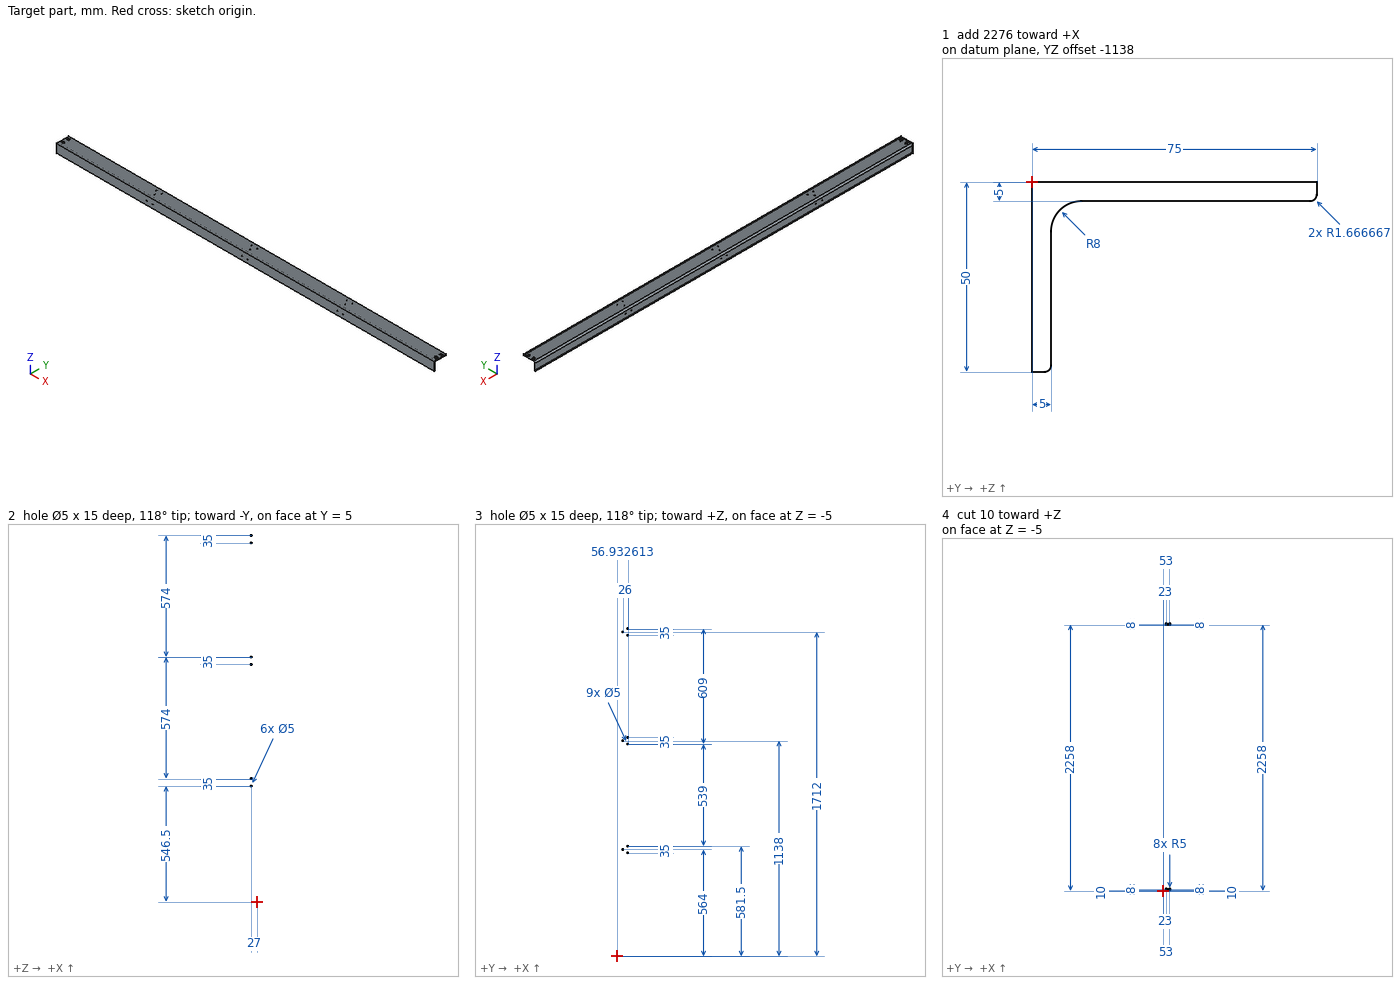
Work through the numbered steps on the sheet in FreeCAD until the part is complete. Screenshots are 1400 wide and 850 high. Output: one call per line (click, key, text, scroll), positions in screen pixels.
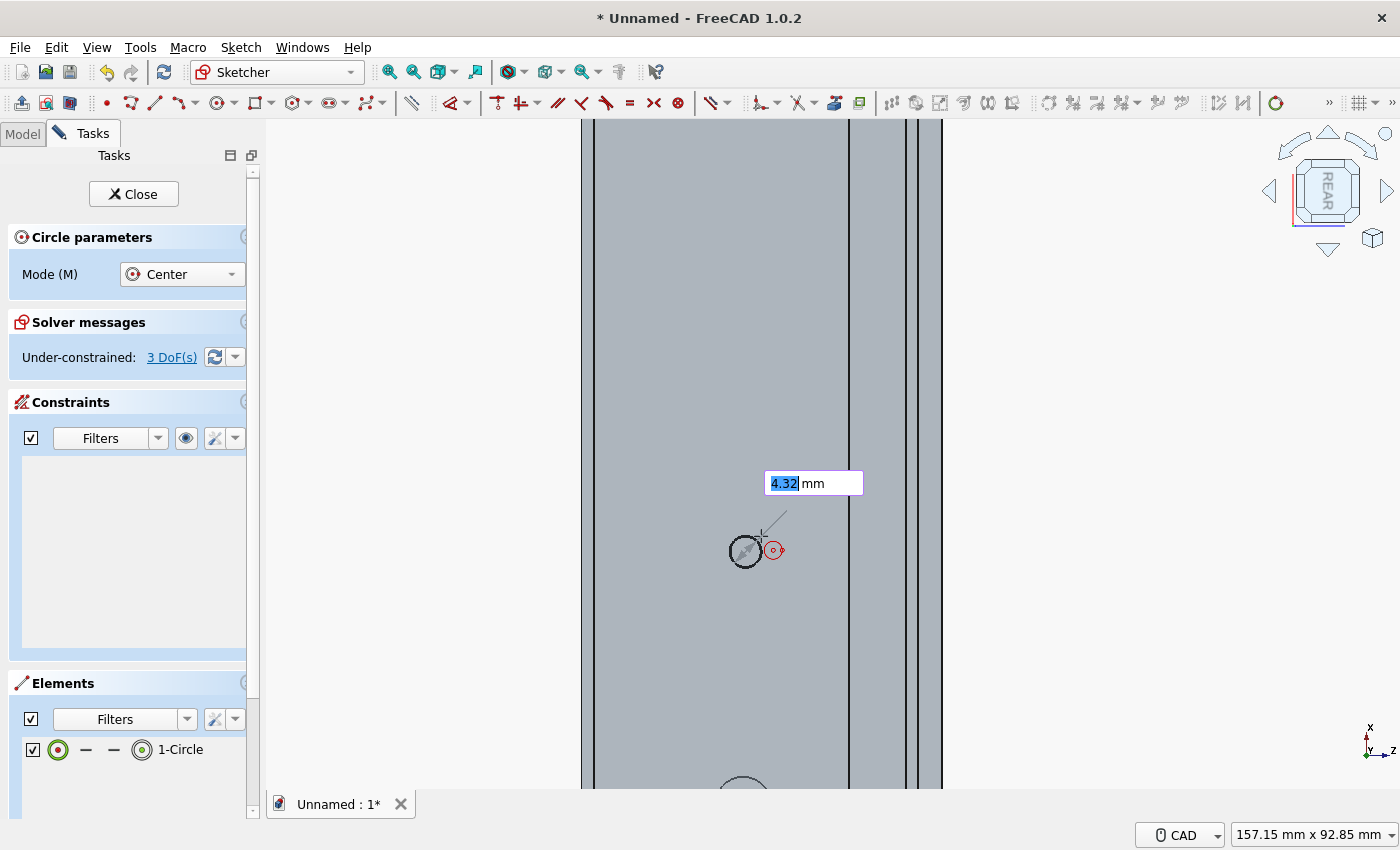
click(760, 530)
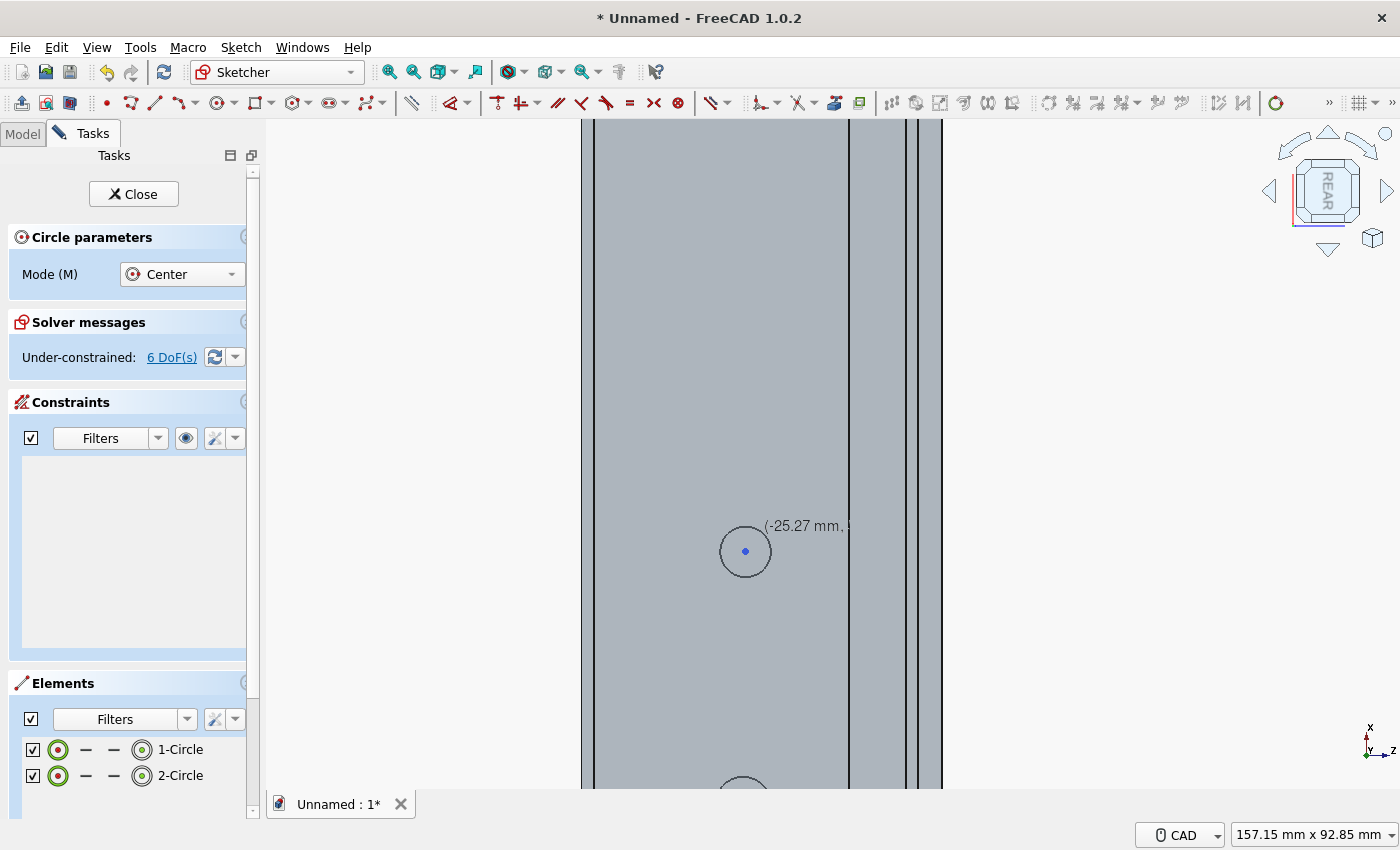
scroll(761, 537, down, 16)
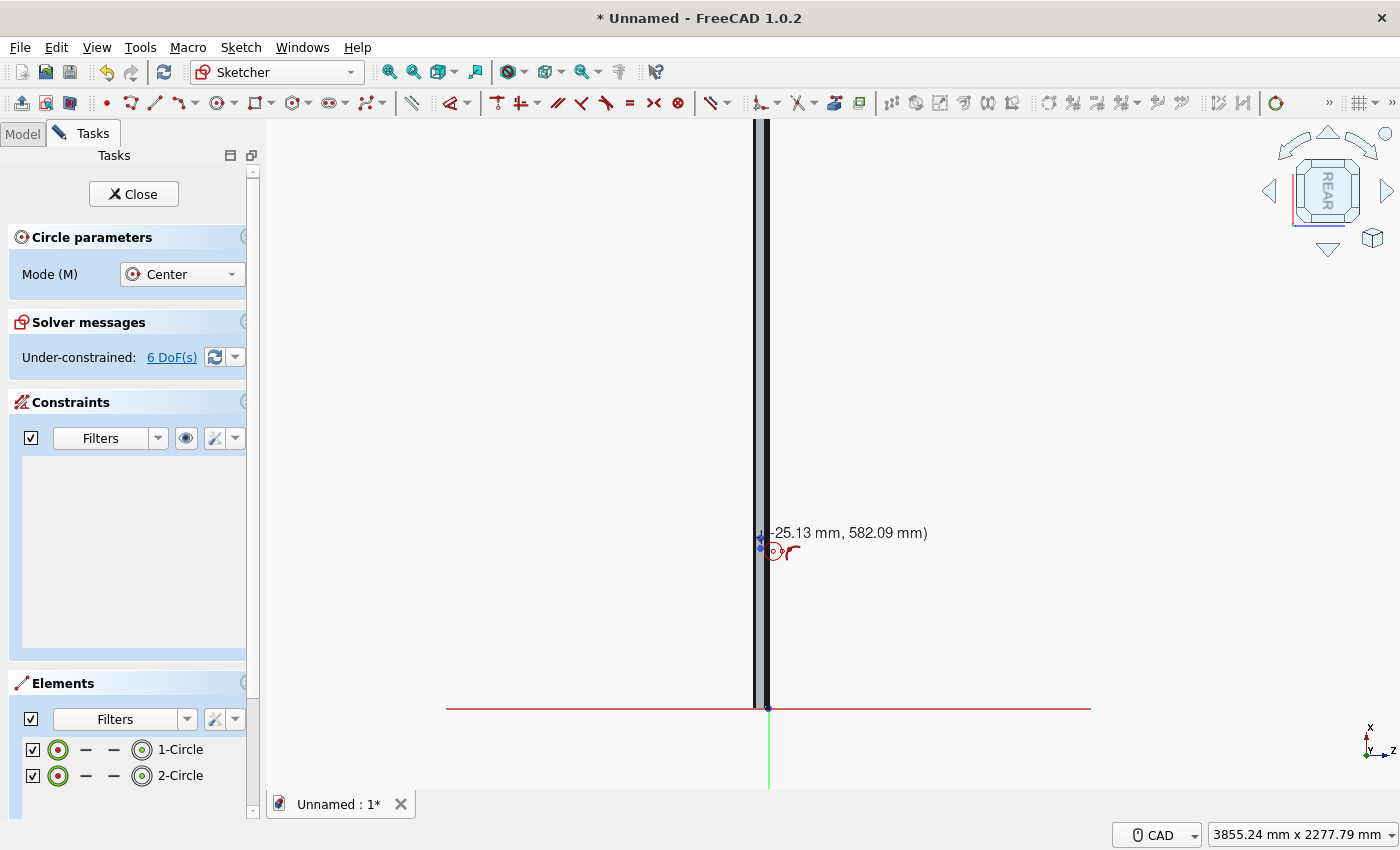
scroll(761, 369, up, 18)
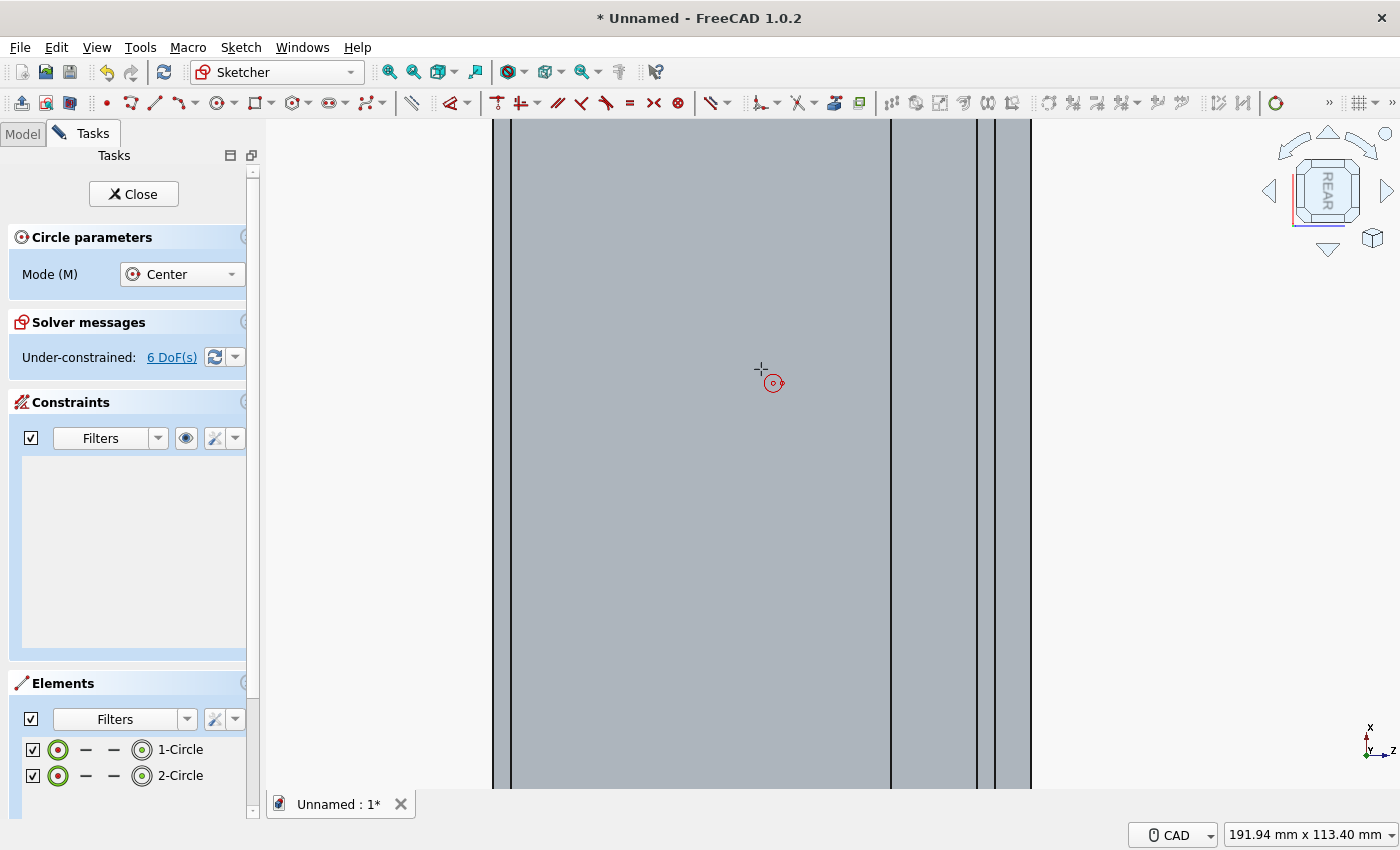
scroll(761, 369, down, 18)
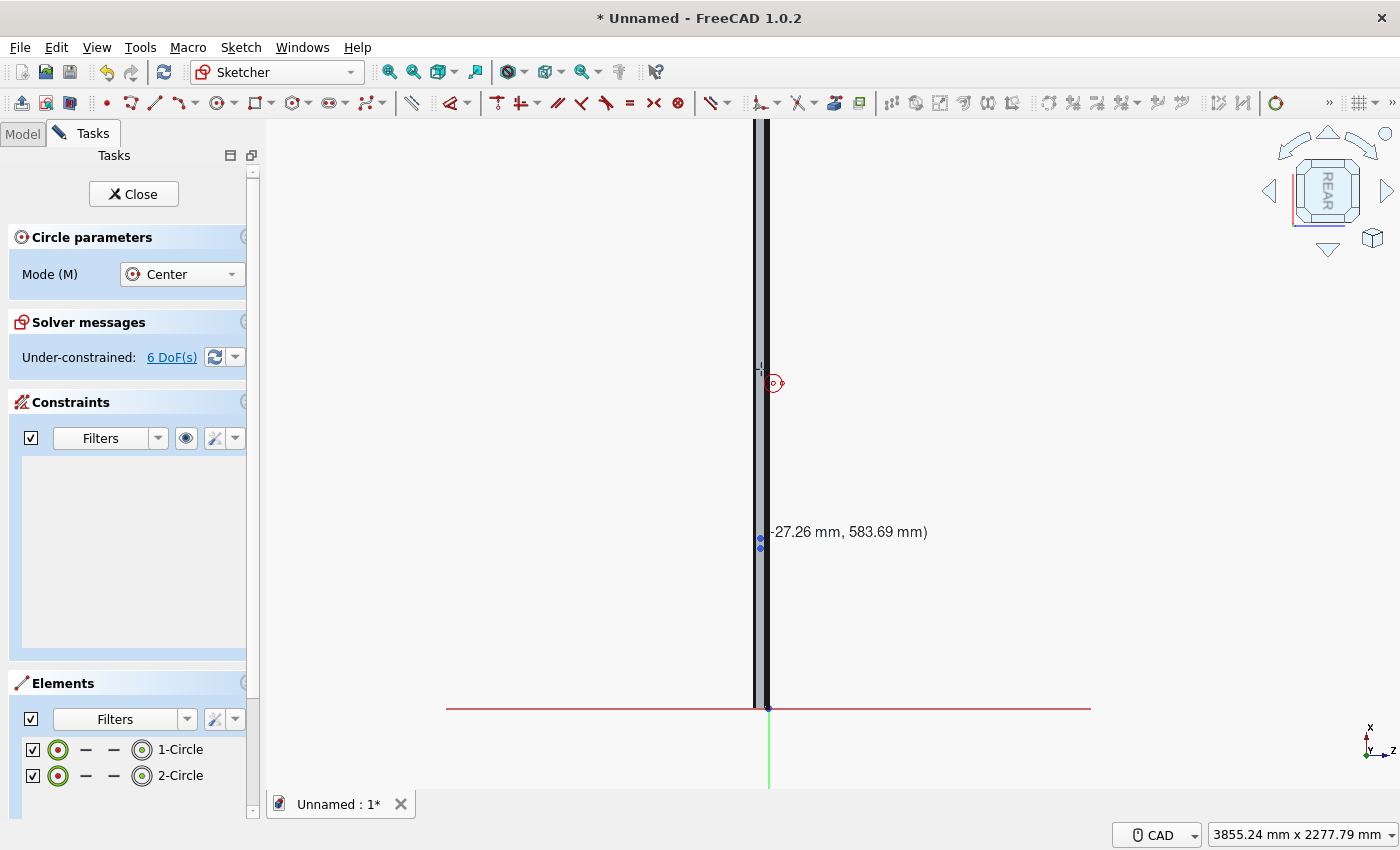
scroll(761, 369, up, 4)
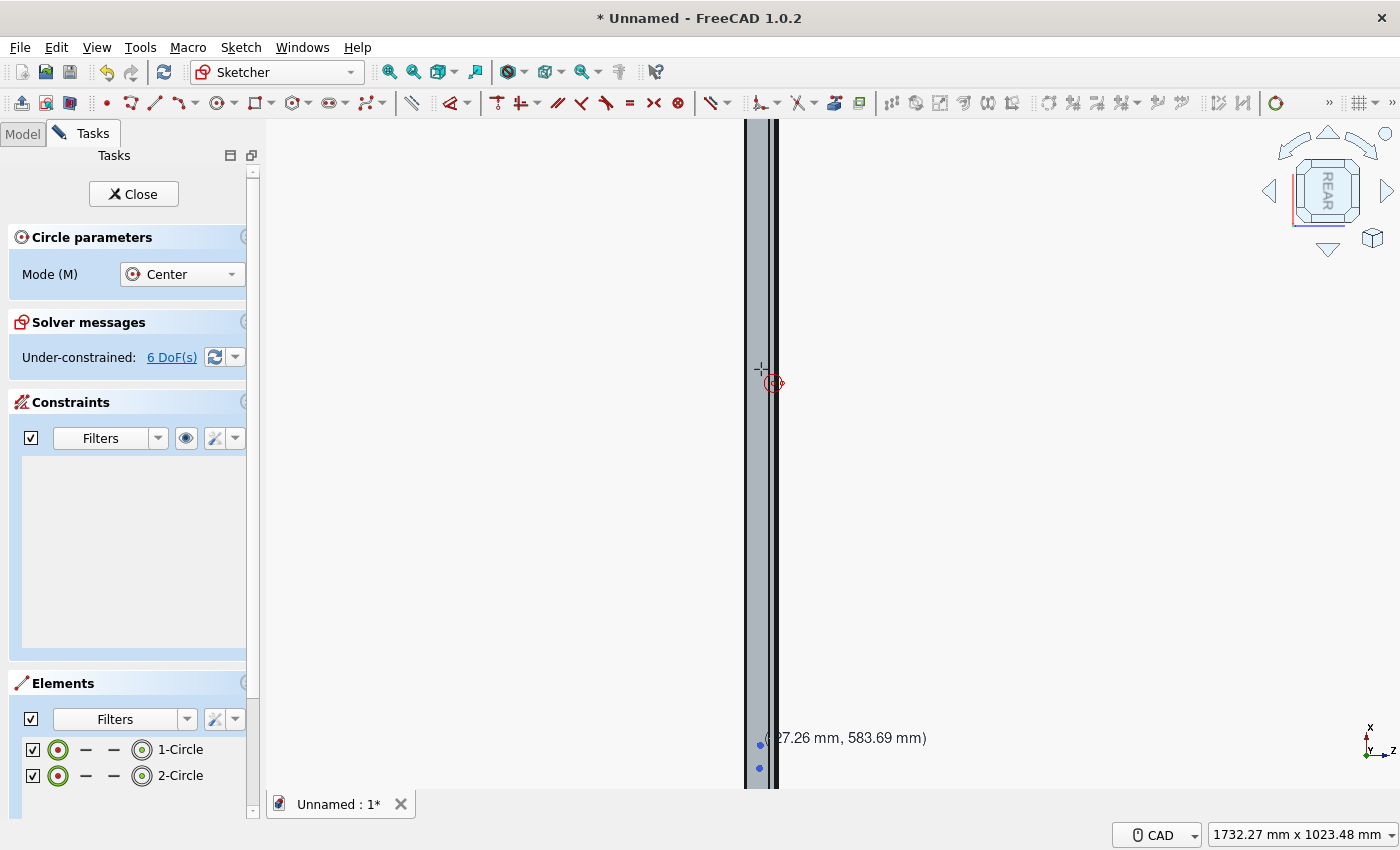
click(760, 368)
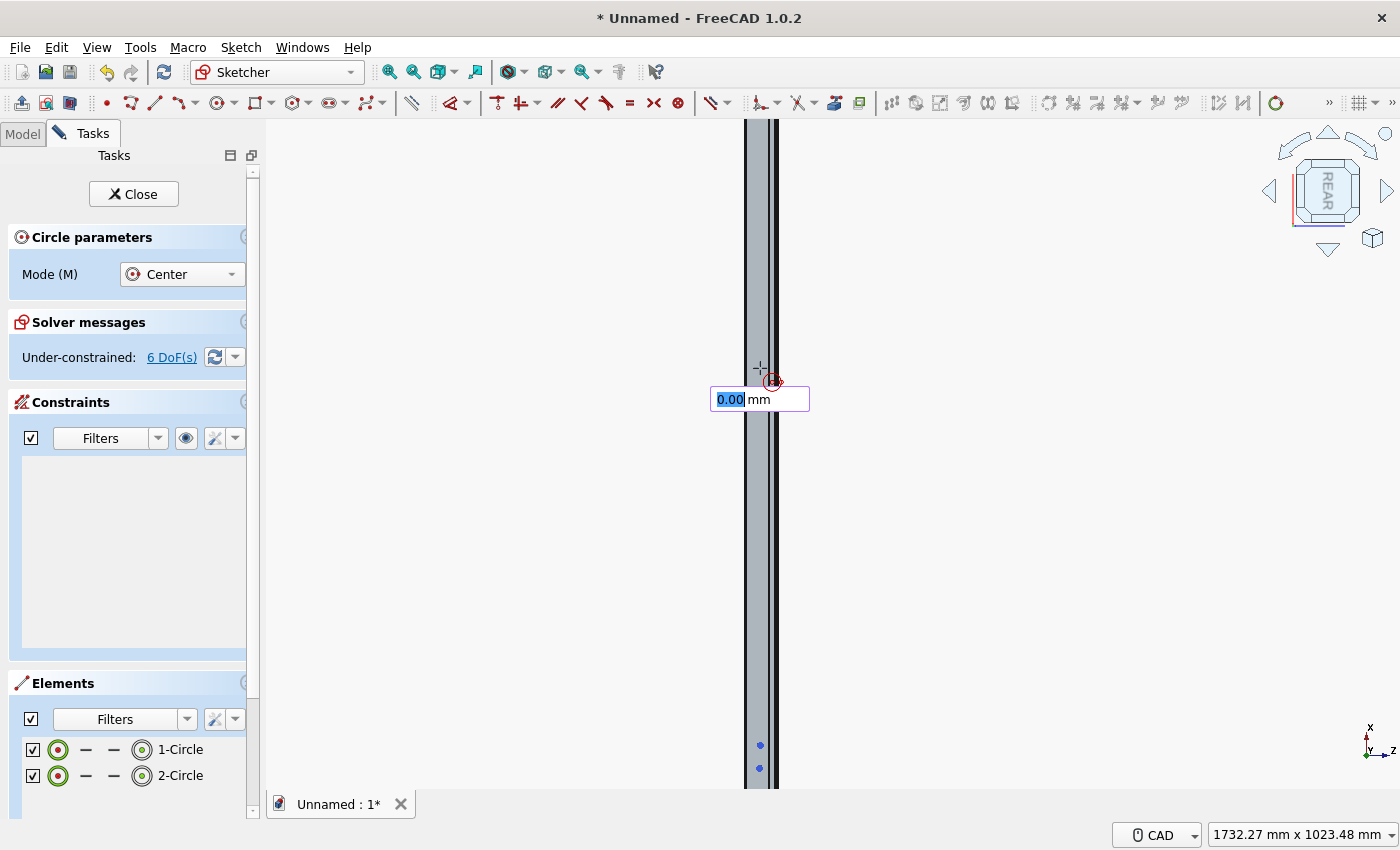
scroll(761, 367, up, 12)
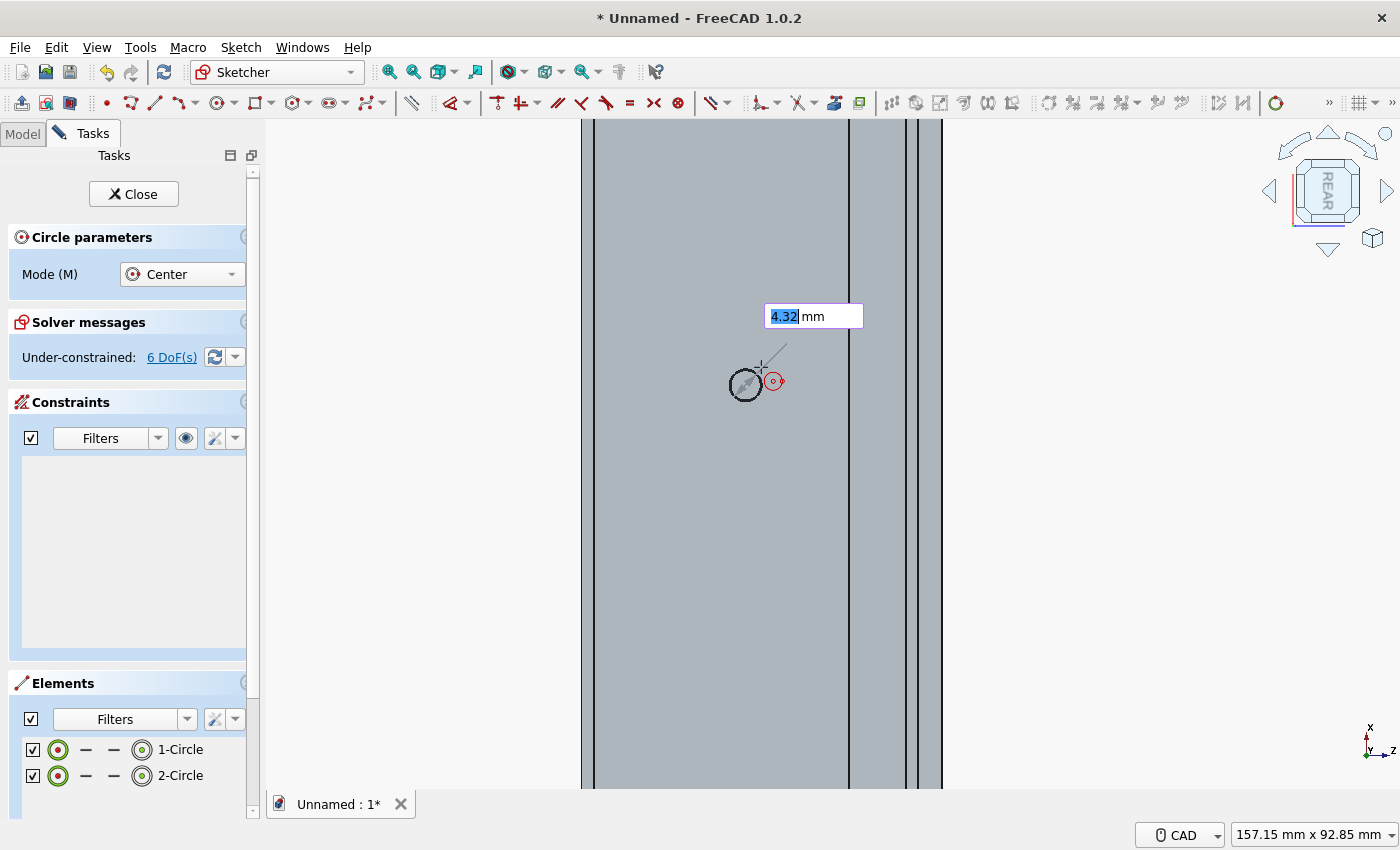
click(760, 367)